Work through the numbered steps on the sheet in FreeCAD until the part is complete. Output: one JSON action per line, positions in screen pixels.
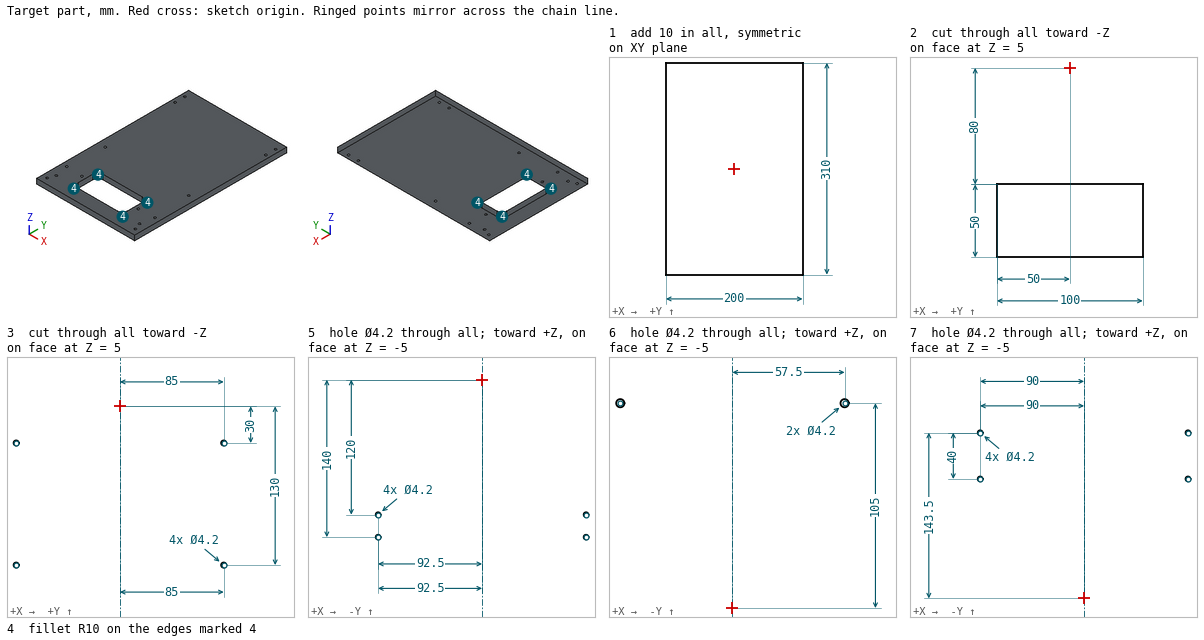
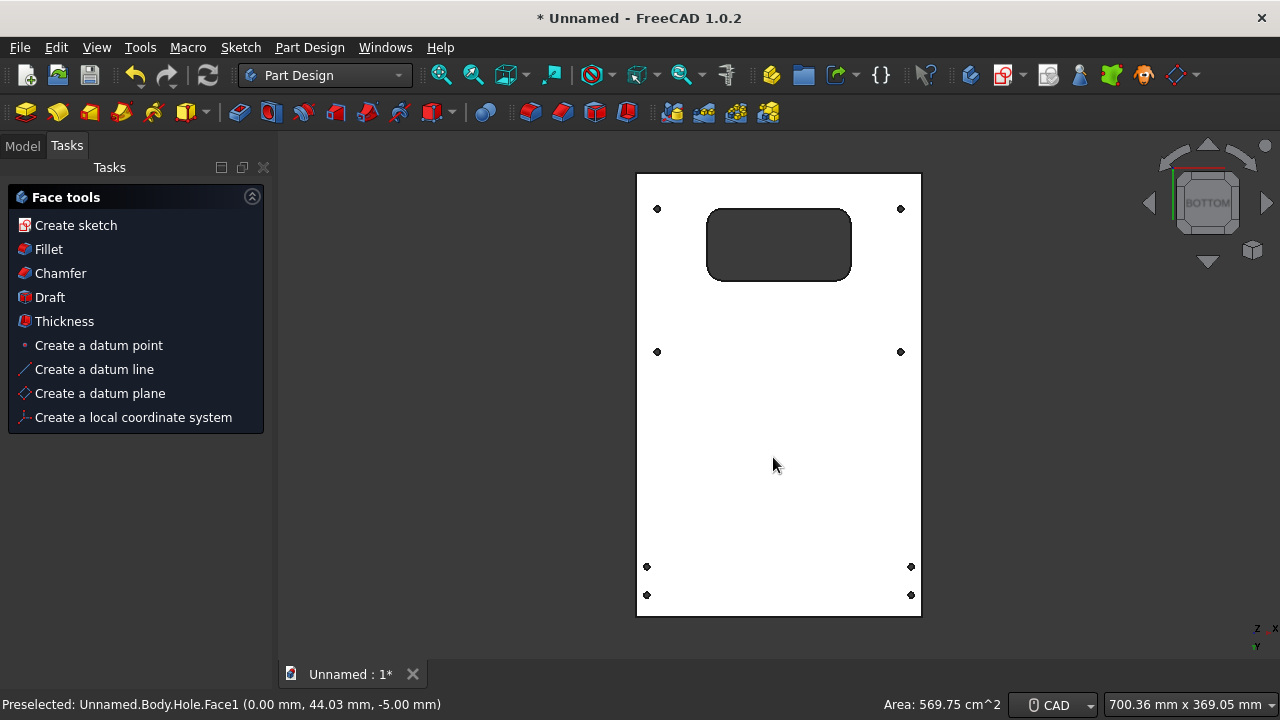
{"action": "left_click", "coordinate": [1004, 76]}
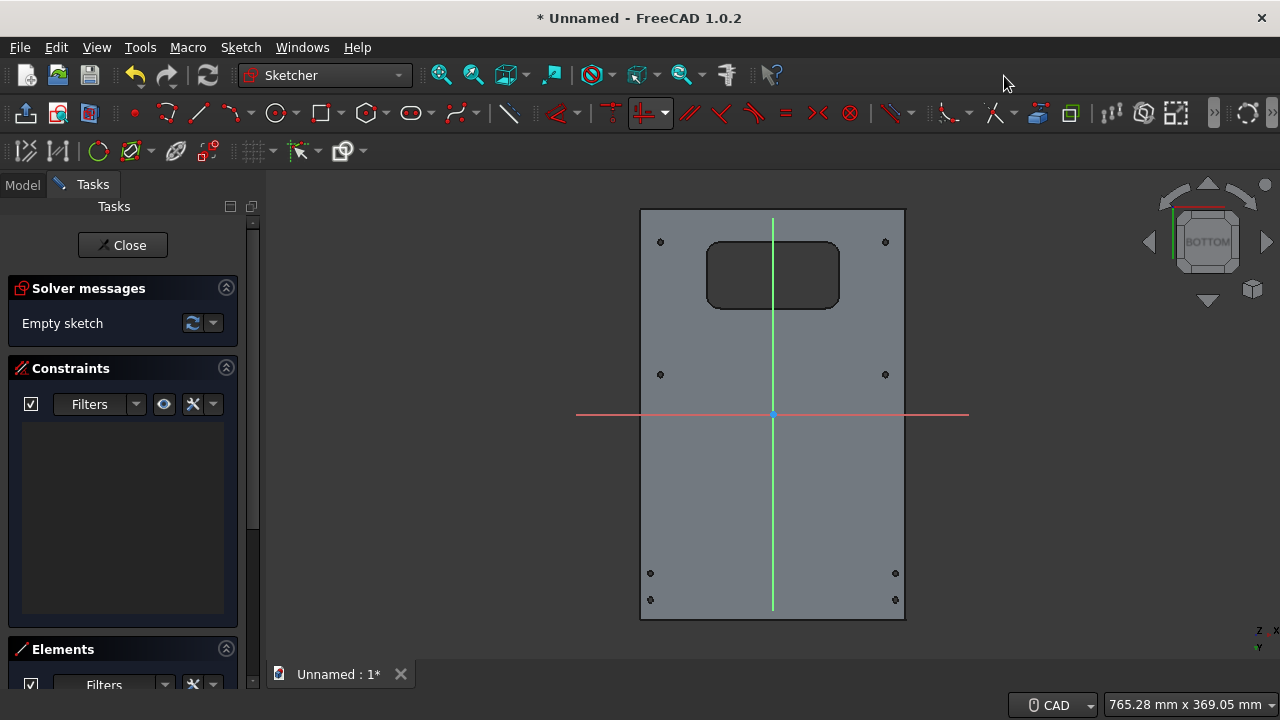
{"action": "scroll", "coordinate": [829, 286], "scroll_direction": "up", "scroll_amount": 4}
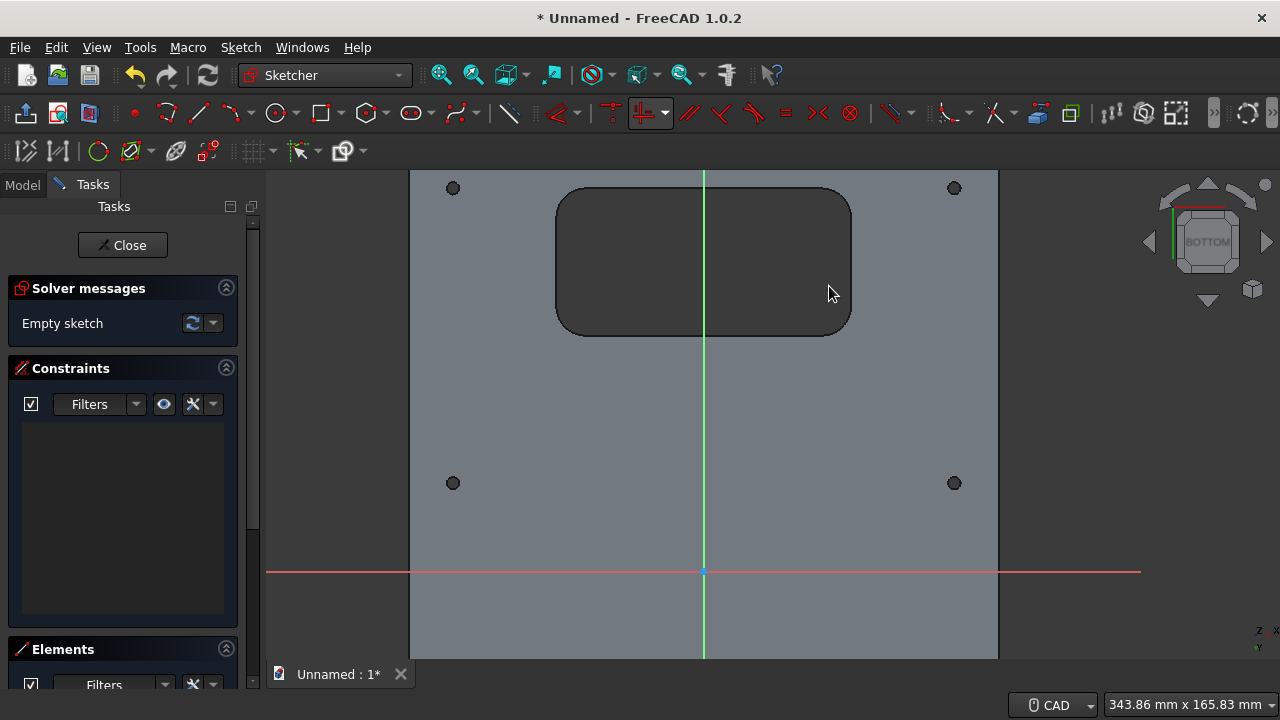
{"action": "left_click", "coordinate": [276, 114]}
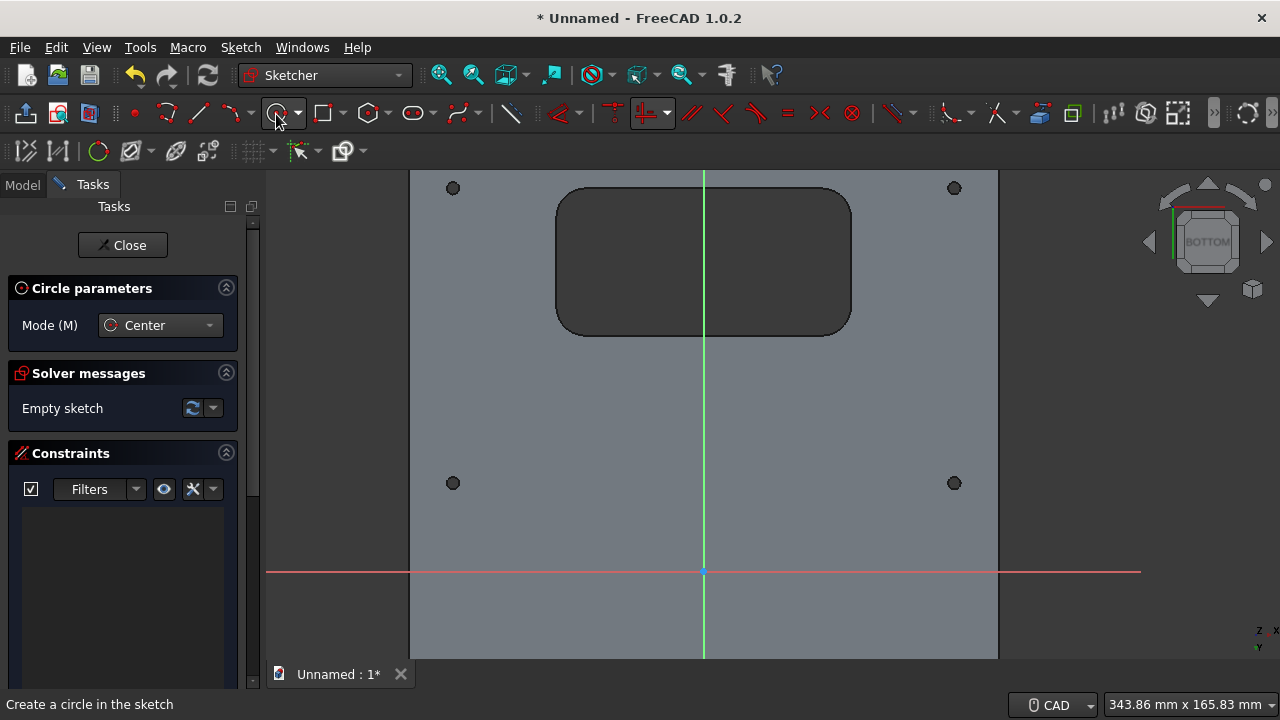
{"action": "scroll", "coordinate": [873, 262], "scroll_direction": "up", "scroll_amount": 7}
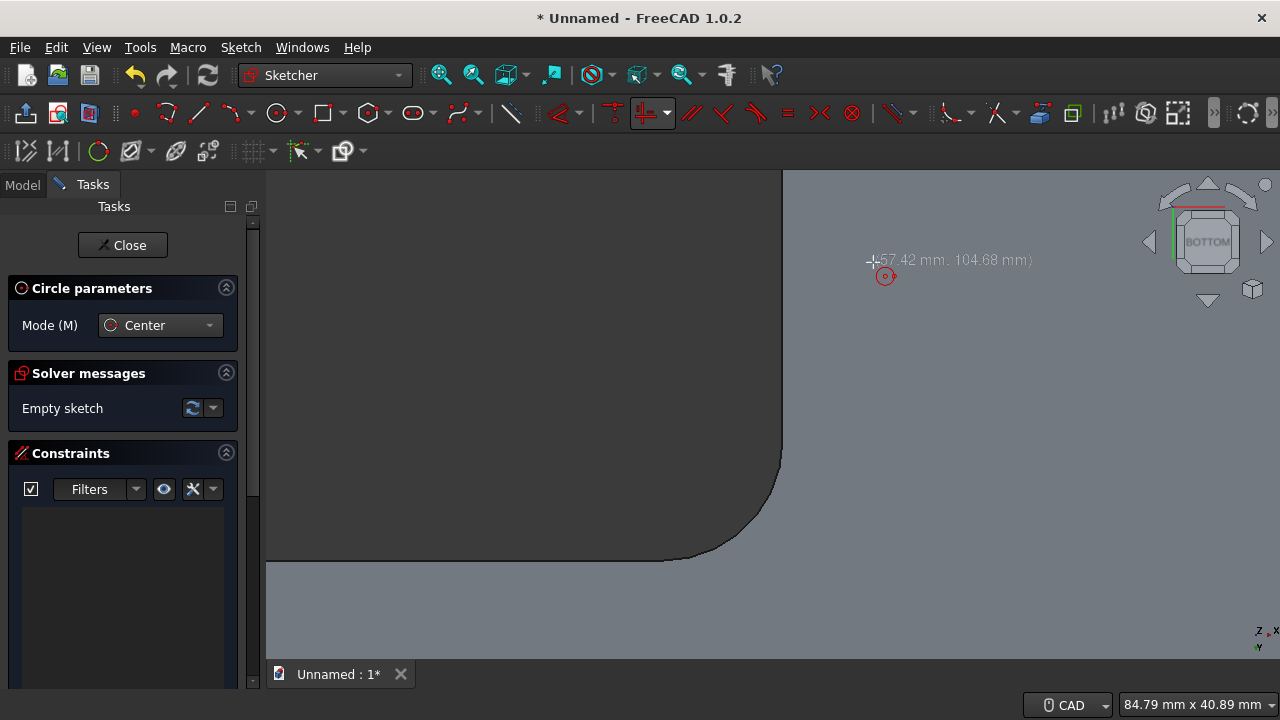
{"action": "scroll", "coordinate": [875, 263], "scroll_direction": "down", "scroll_amount": 7}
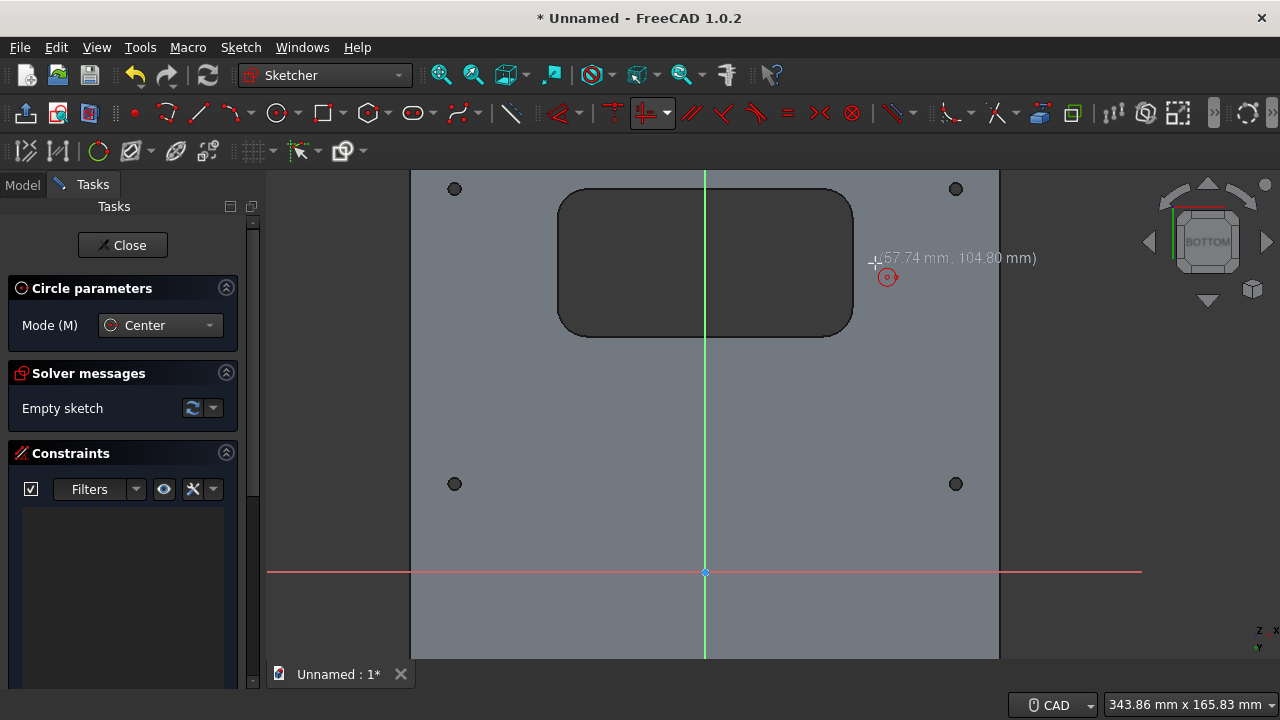
{"action": "left_click", "coordinate": [875, 263]}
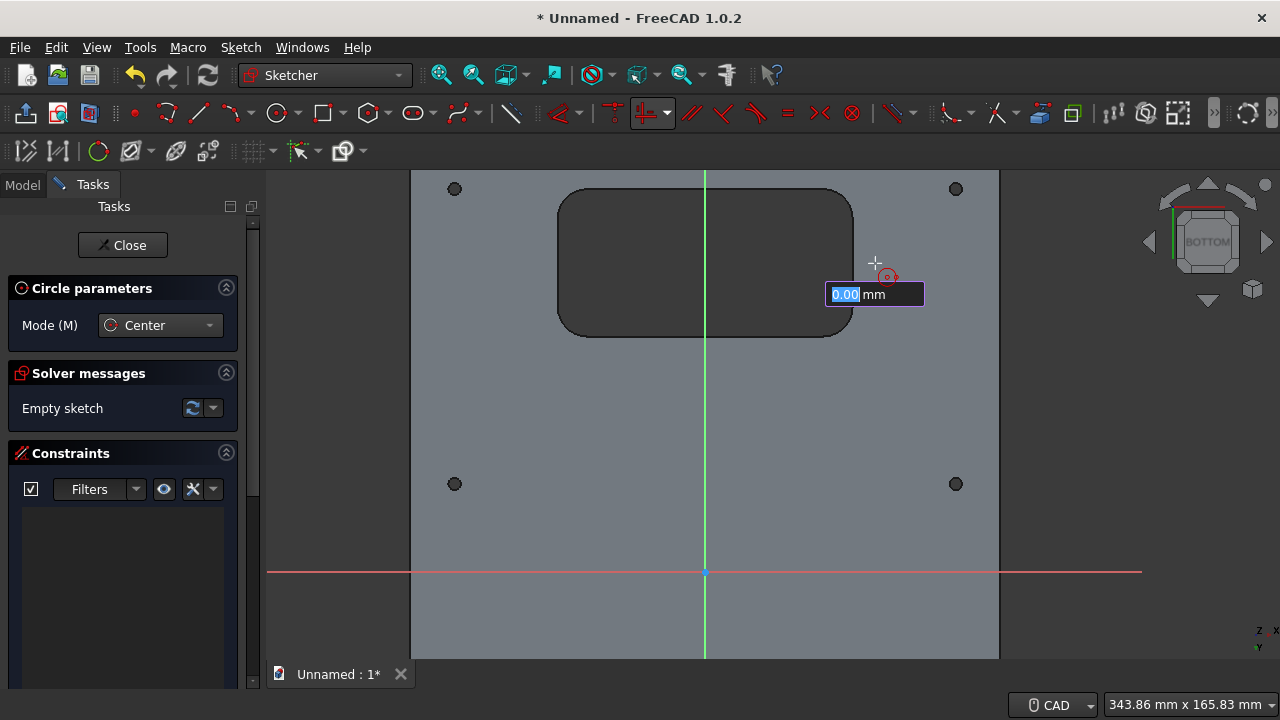
{"action": "scroll", "coordinate": [879, 258], "scroll_direction": "up", "scroll_amount": 5}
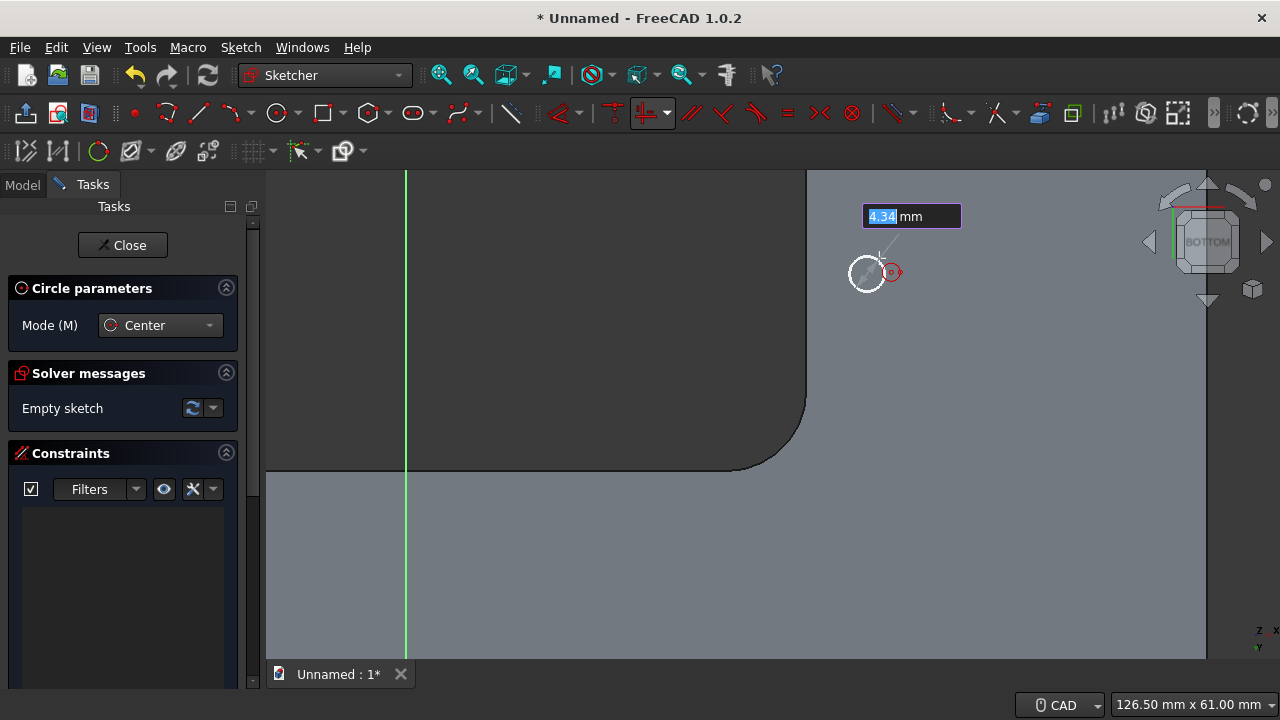
{"action": "left_click", "coordinate": [878, 259]}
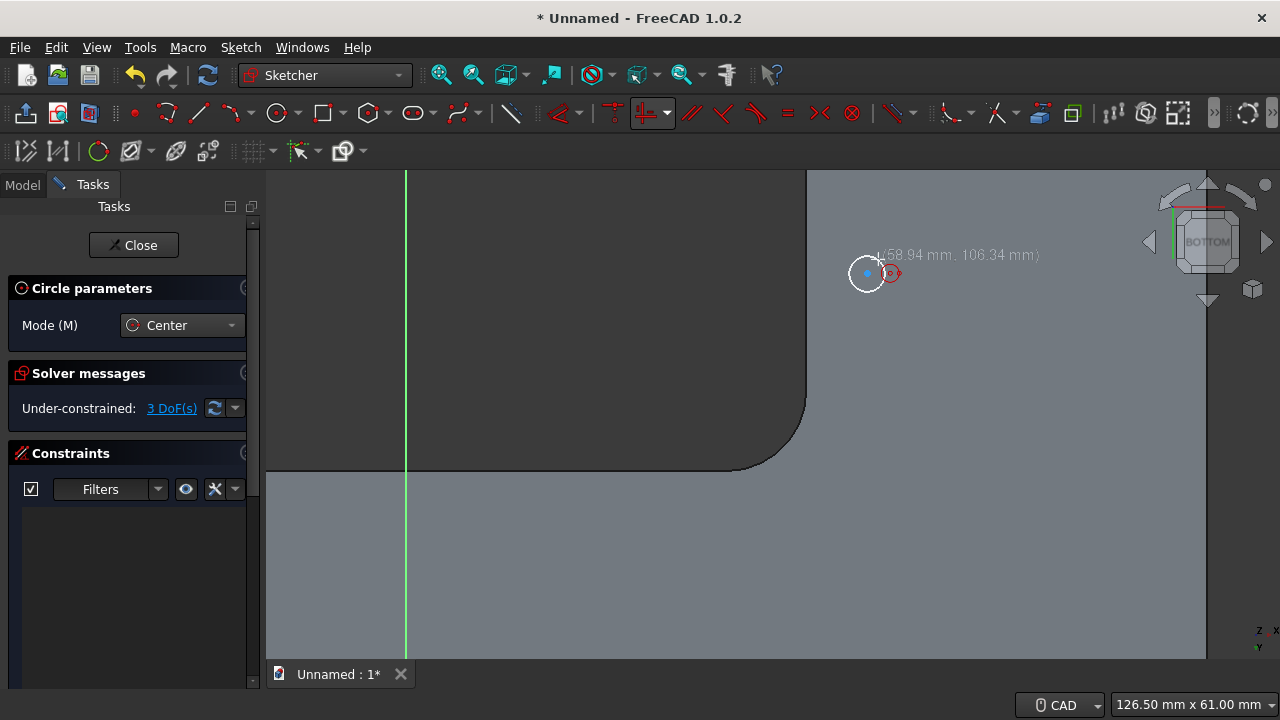
{"action": "scroll", "coordinate": [879, 258], "scroll_direction": "down", "scroll_amount": 5}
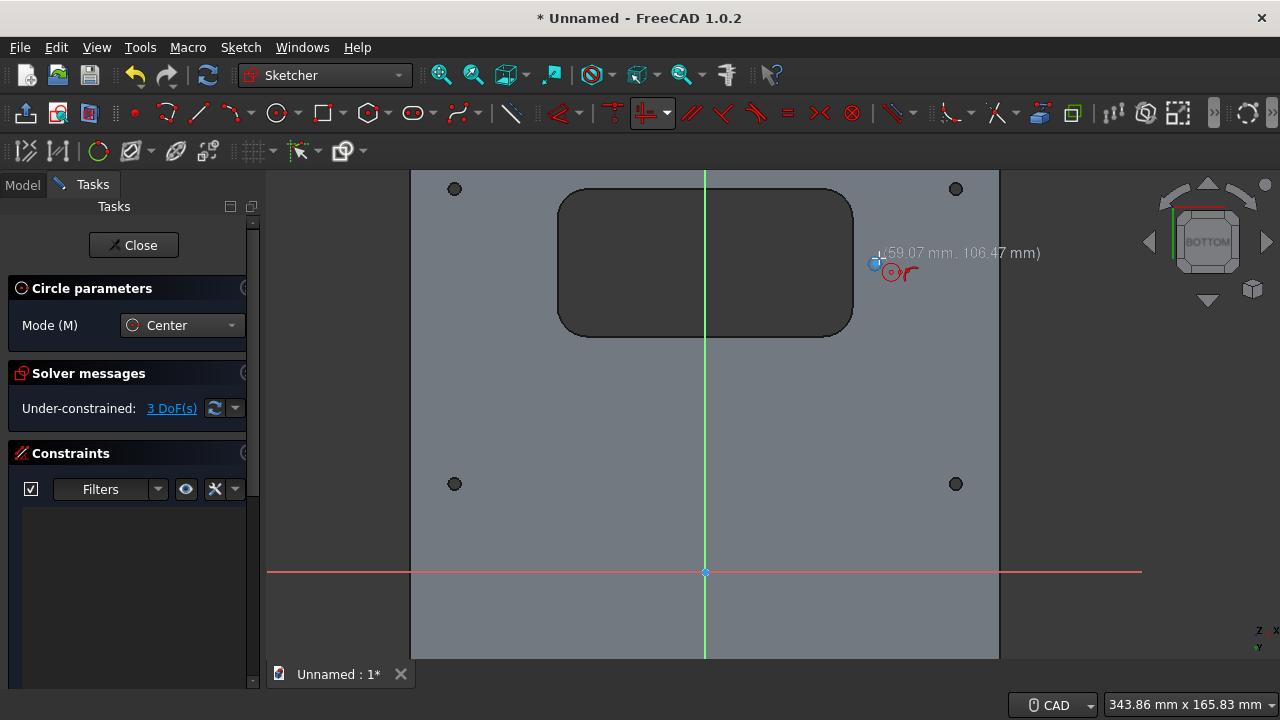
{"action": "scroll", "coordinate": [536, 263], "scroll_direction": "up", "scroll_amount": 7}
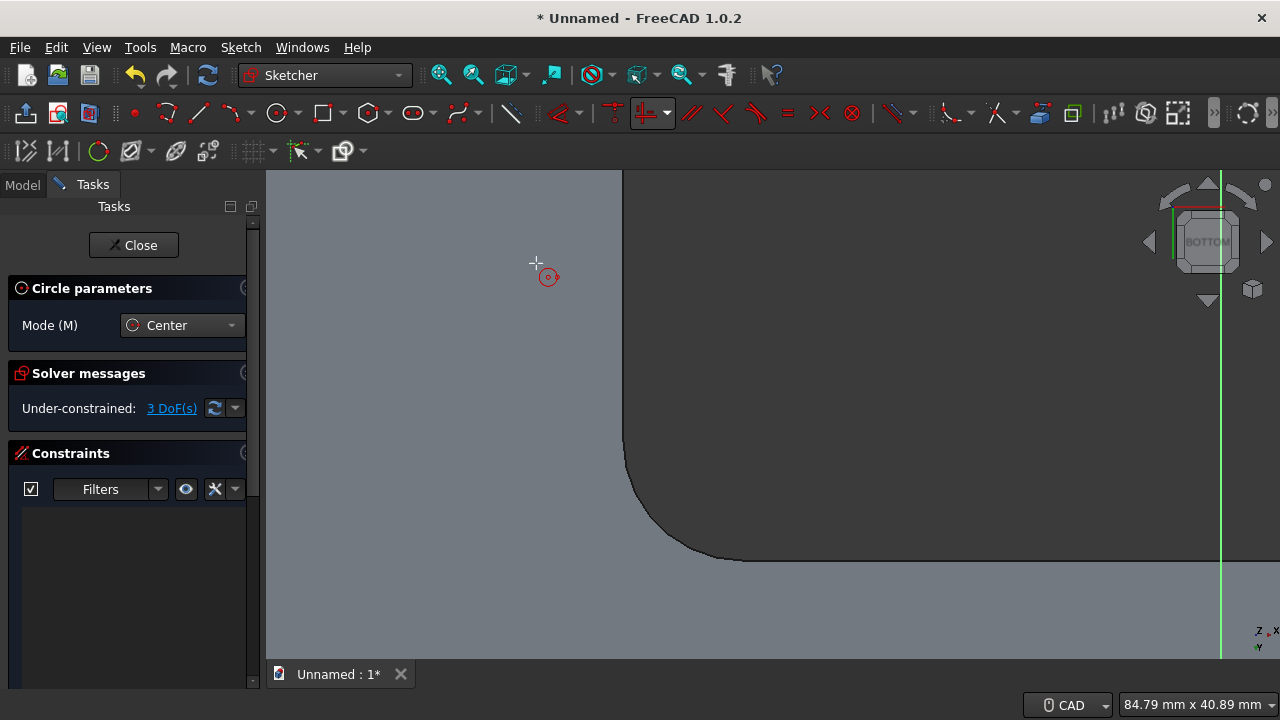
{"action": "scroll", "coordinate": [535, 263], "scroll_direction": "down", "scroll_amount": 7}